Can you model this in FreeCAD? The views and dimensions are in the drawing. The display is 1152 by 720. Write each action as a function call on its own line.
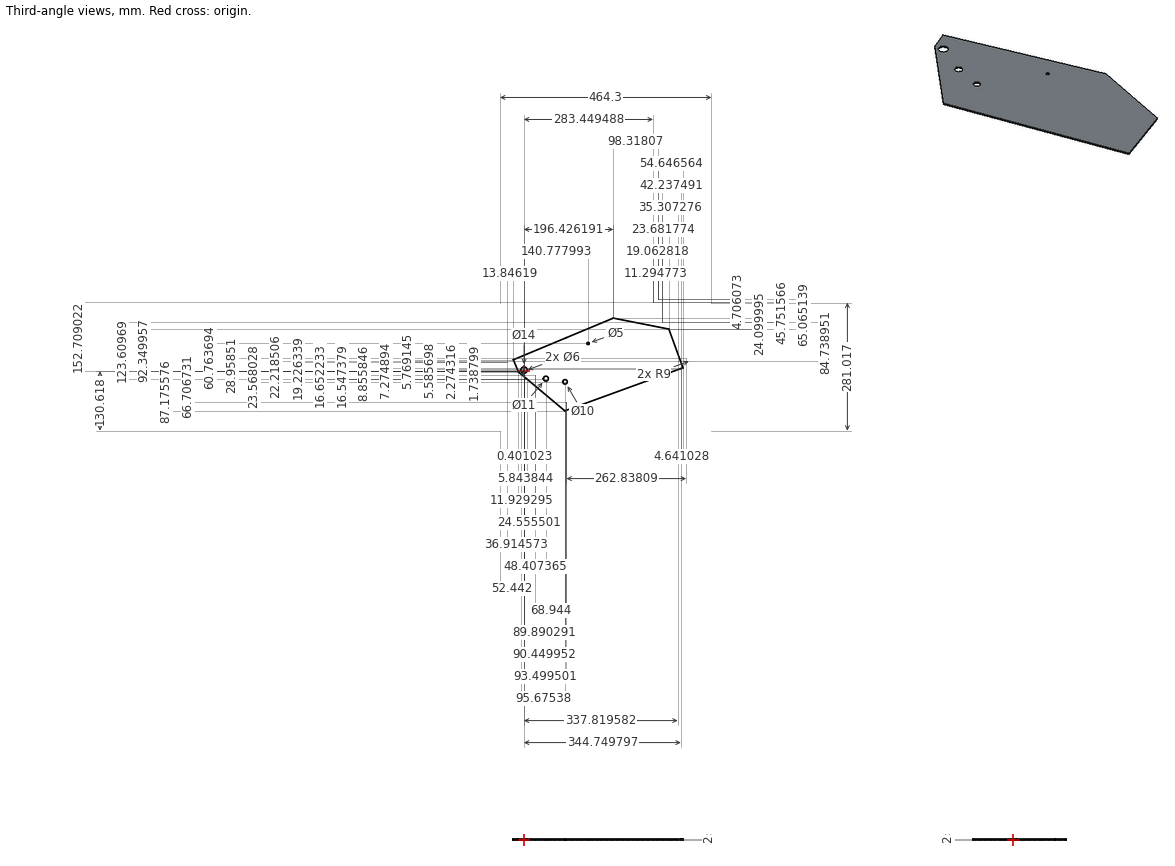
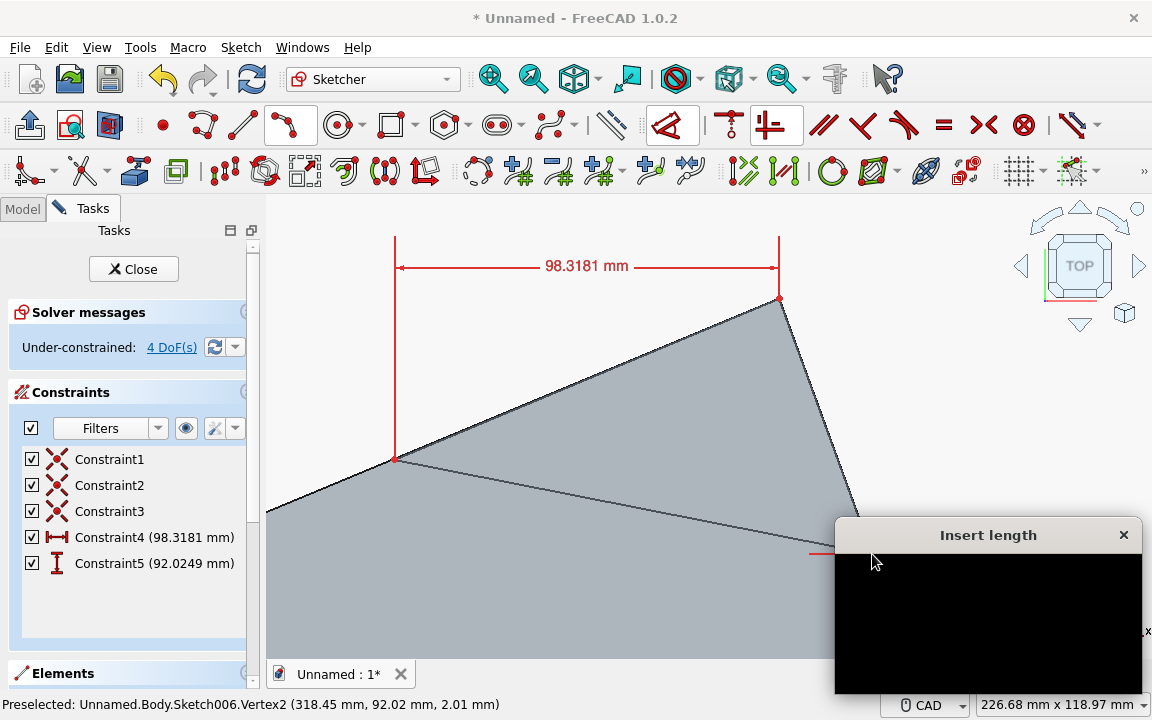
text(92.349957)
key(Return)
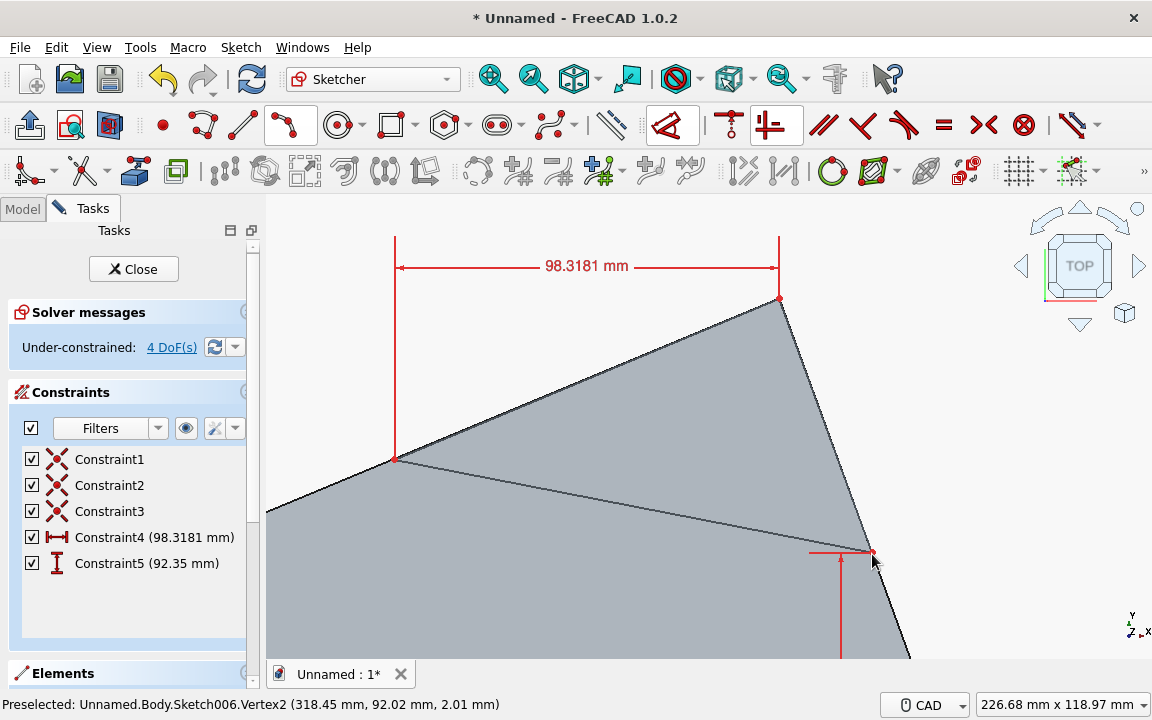
click(538, 488)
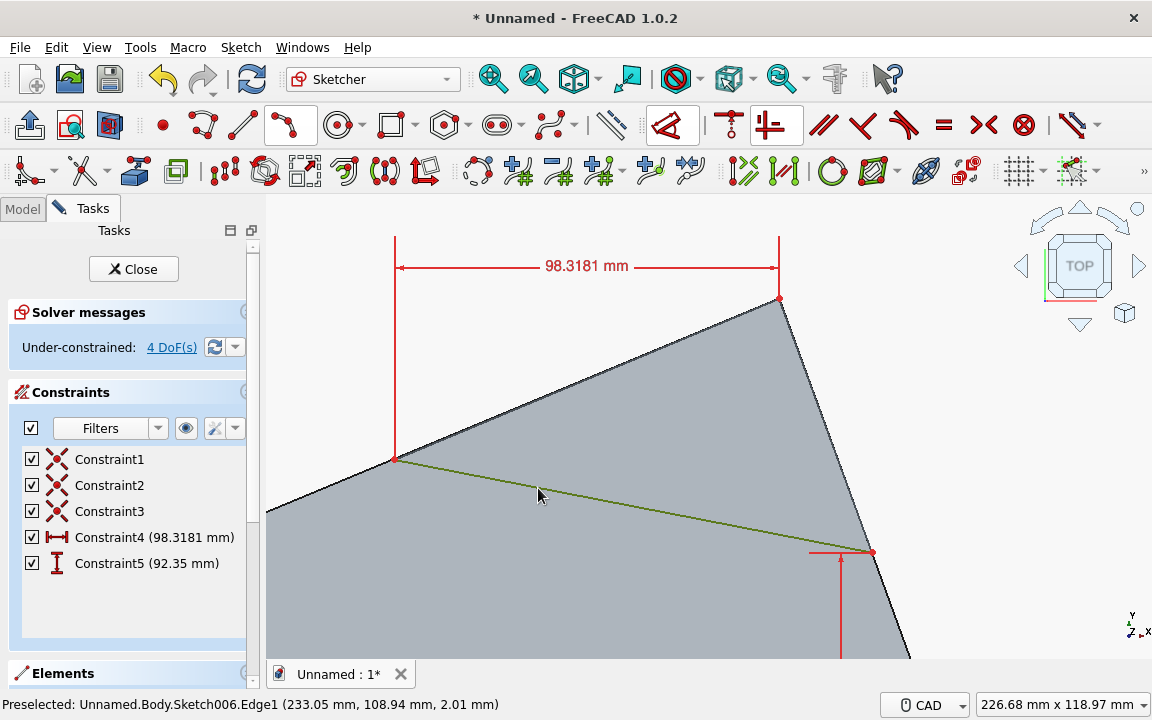
key(i)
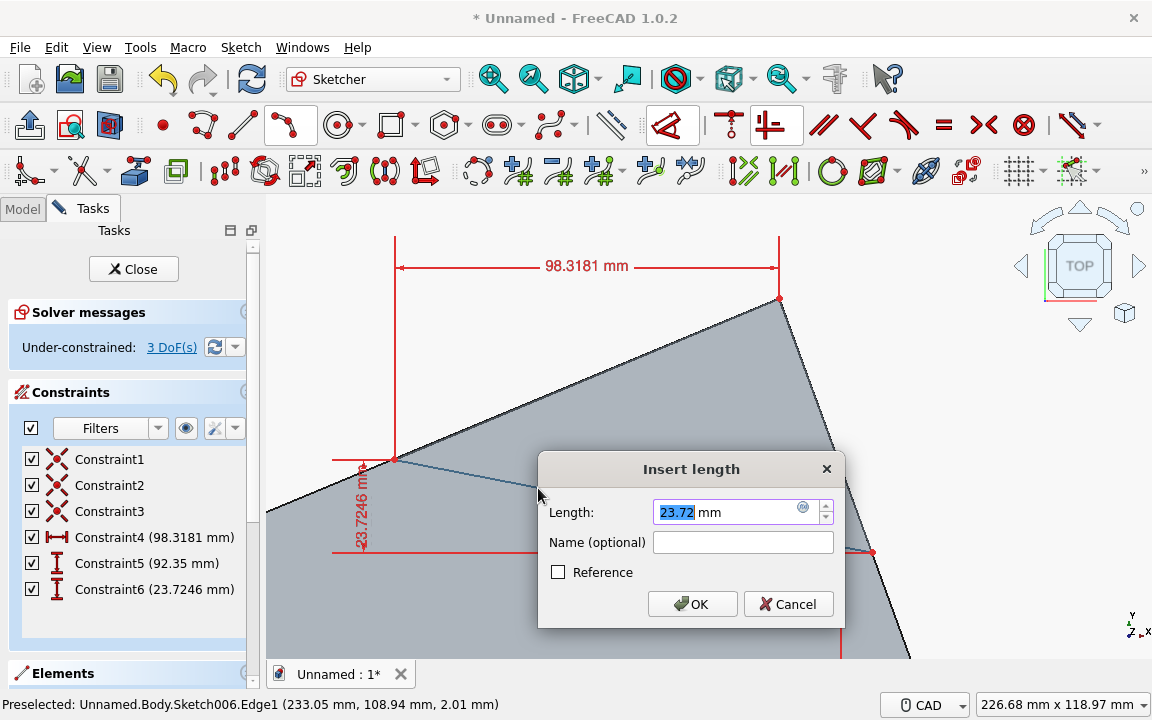
text(24.099995)
key(Return)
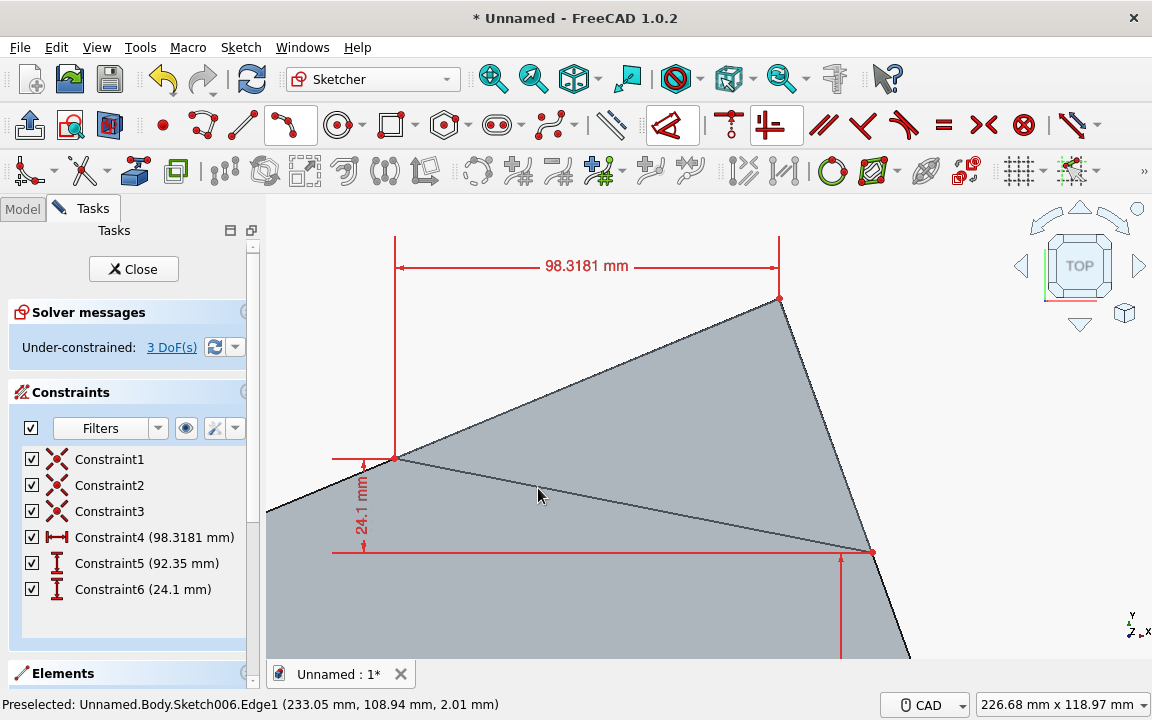
click(844, 477)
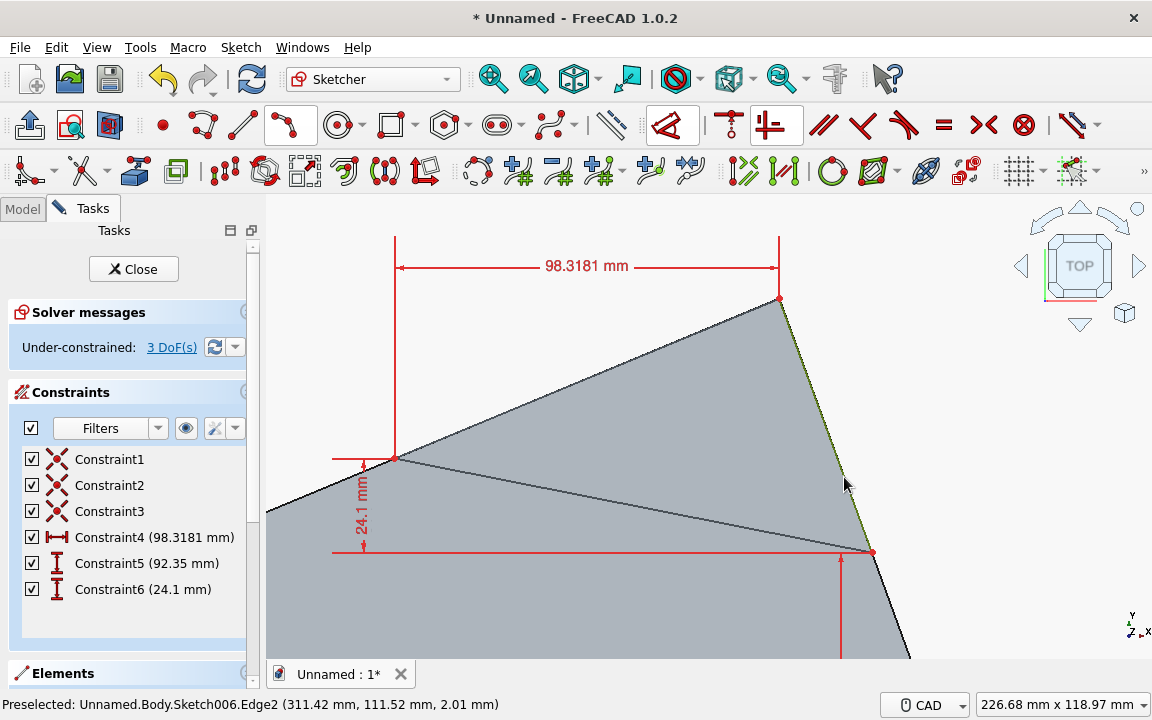
key(l)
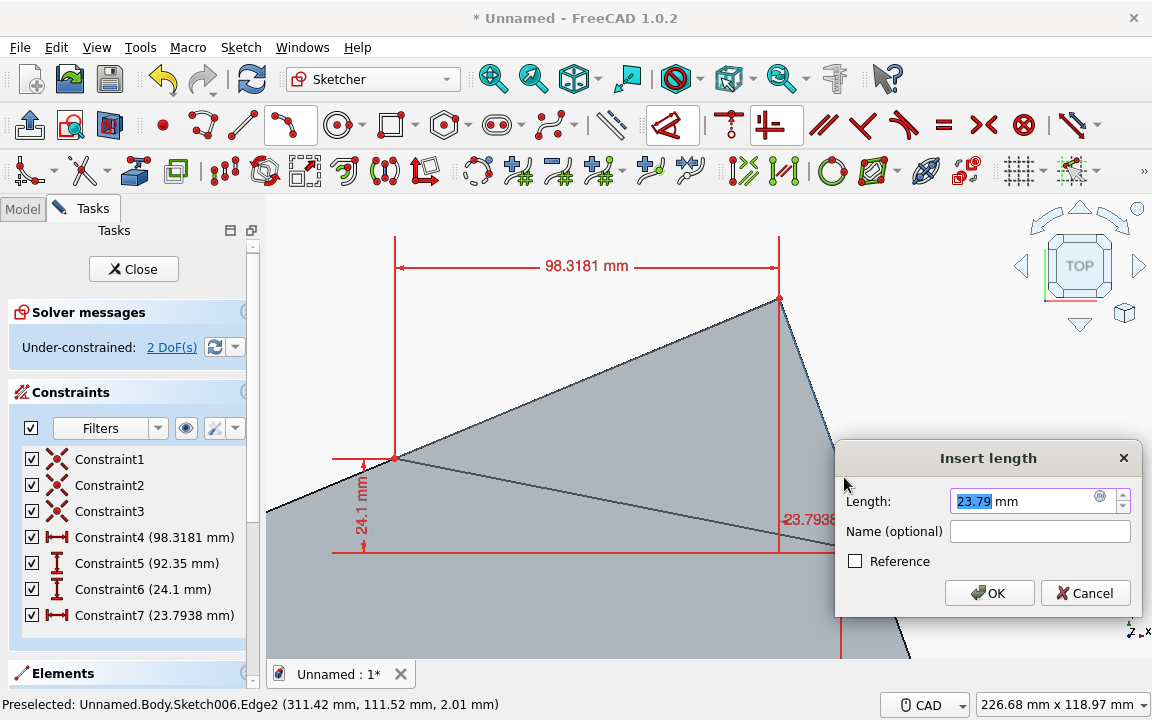
text(23.681774)
key(Return)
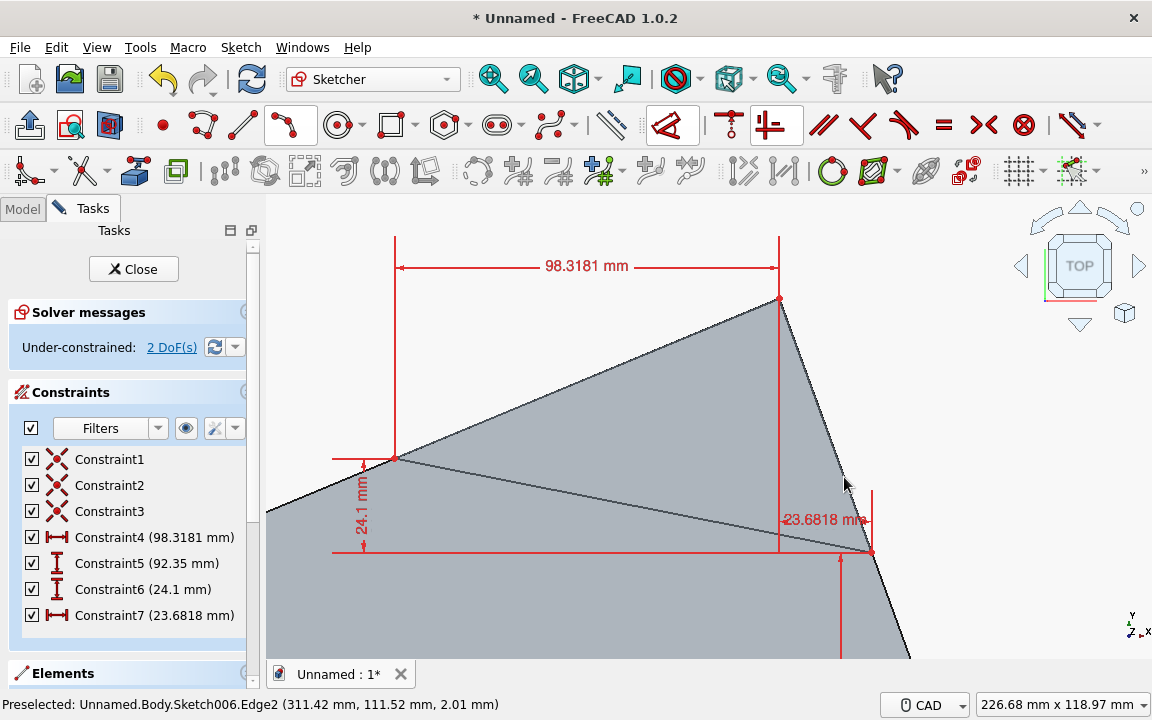
click(844, 477)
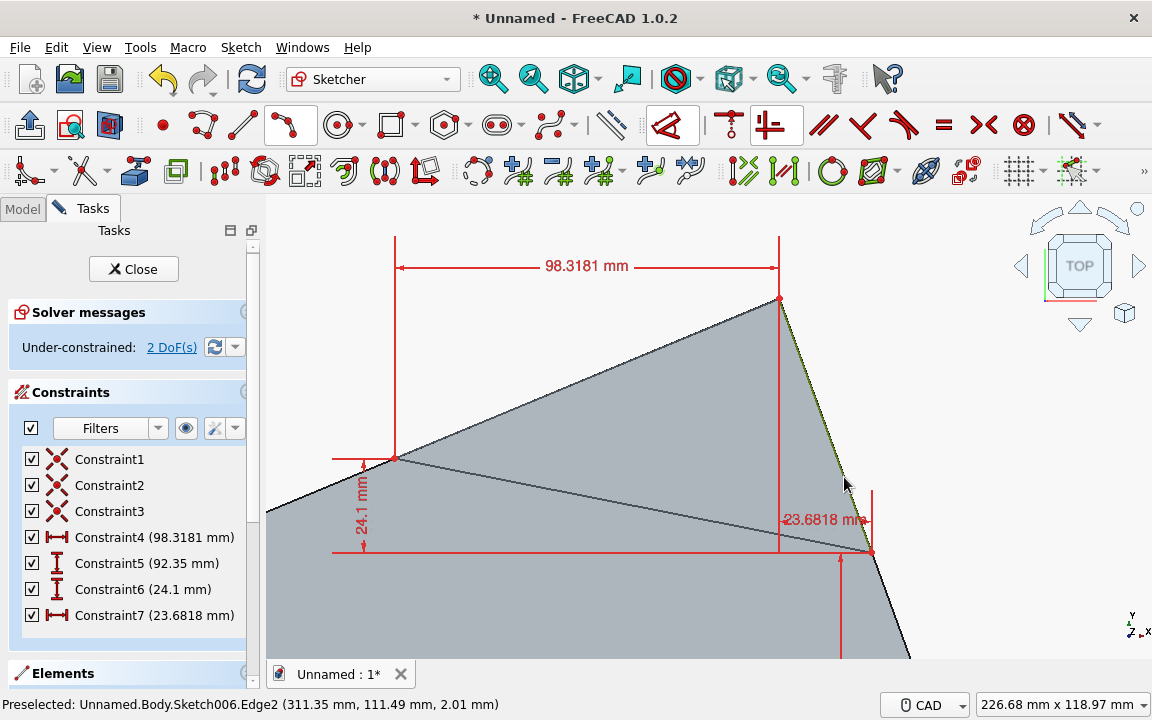
key(i)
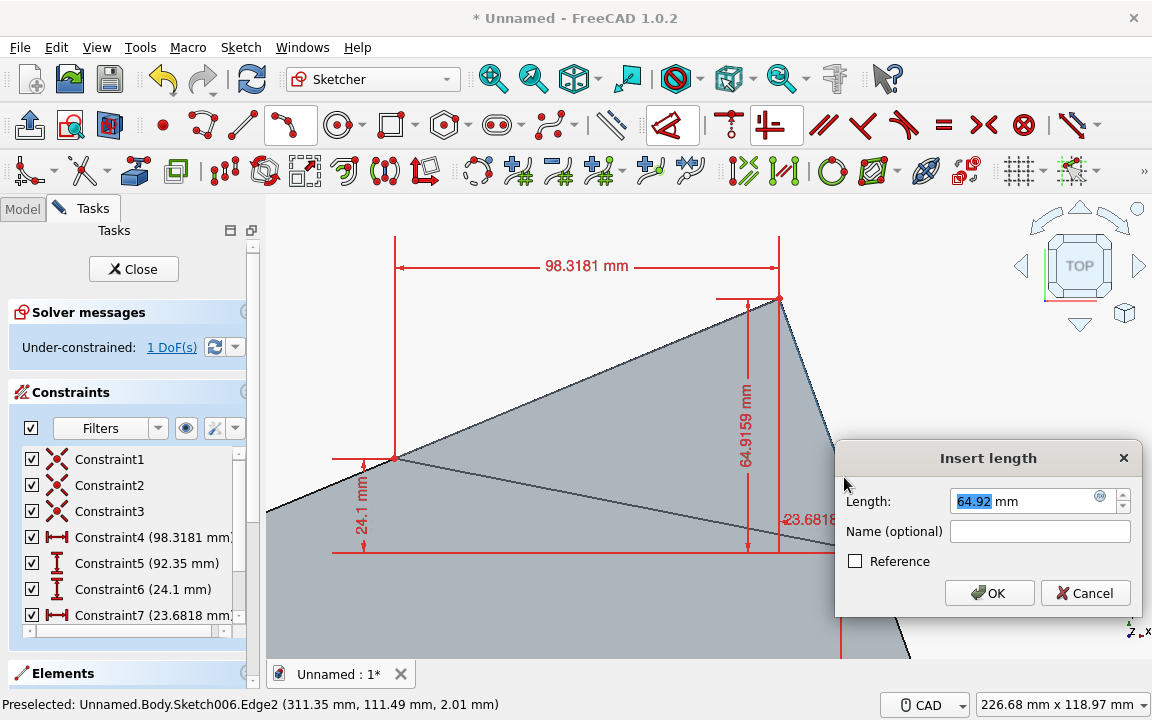
text(65.065139)
key(Return)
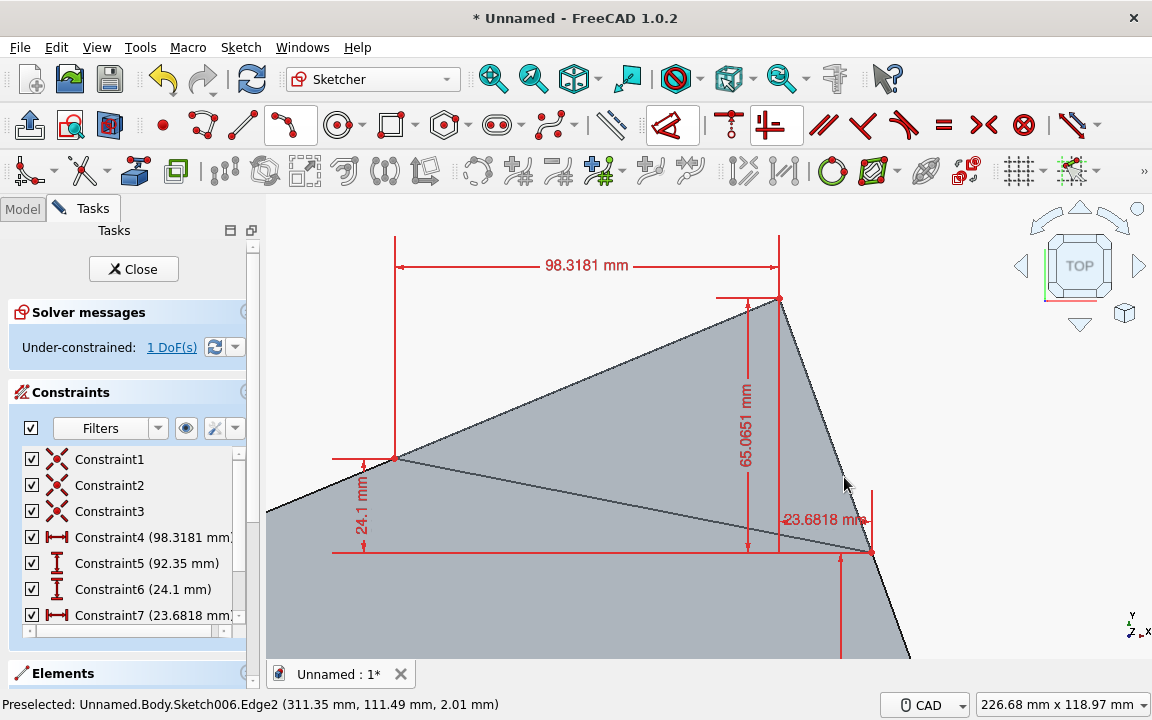
click(395, 459)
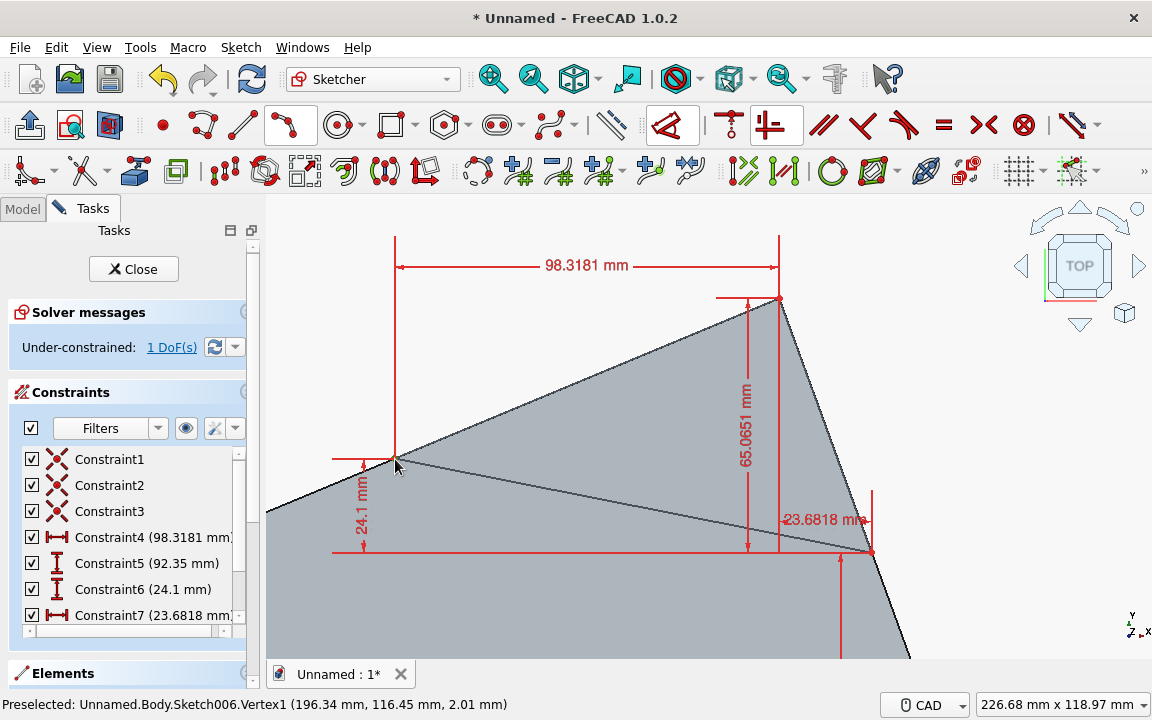
key(l)